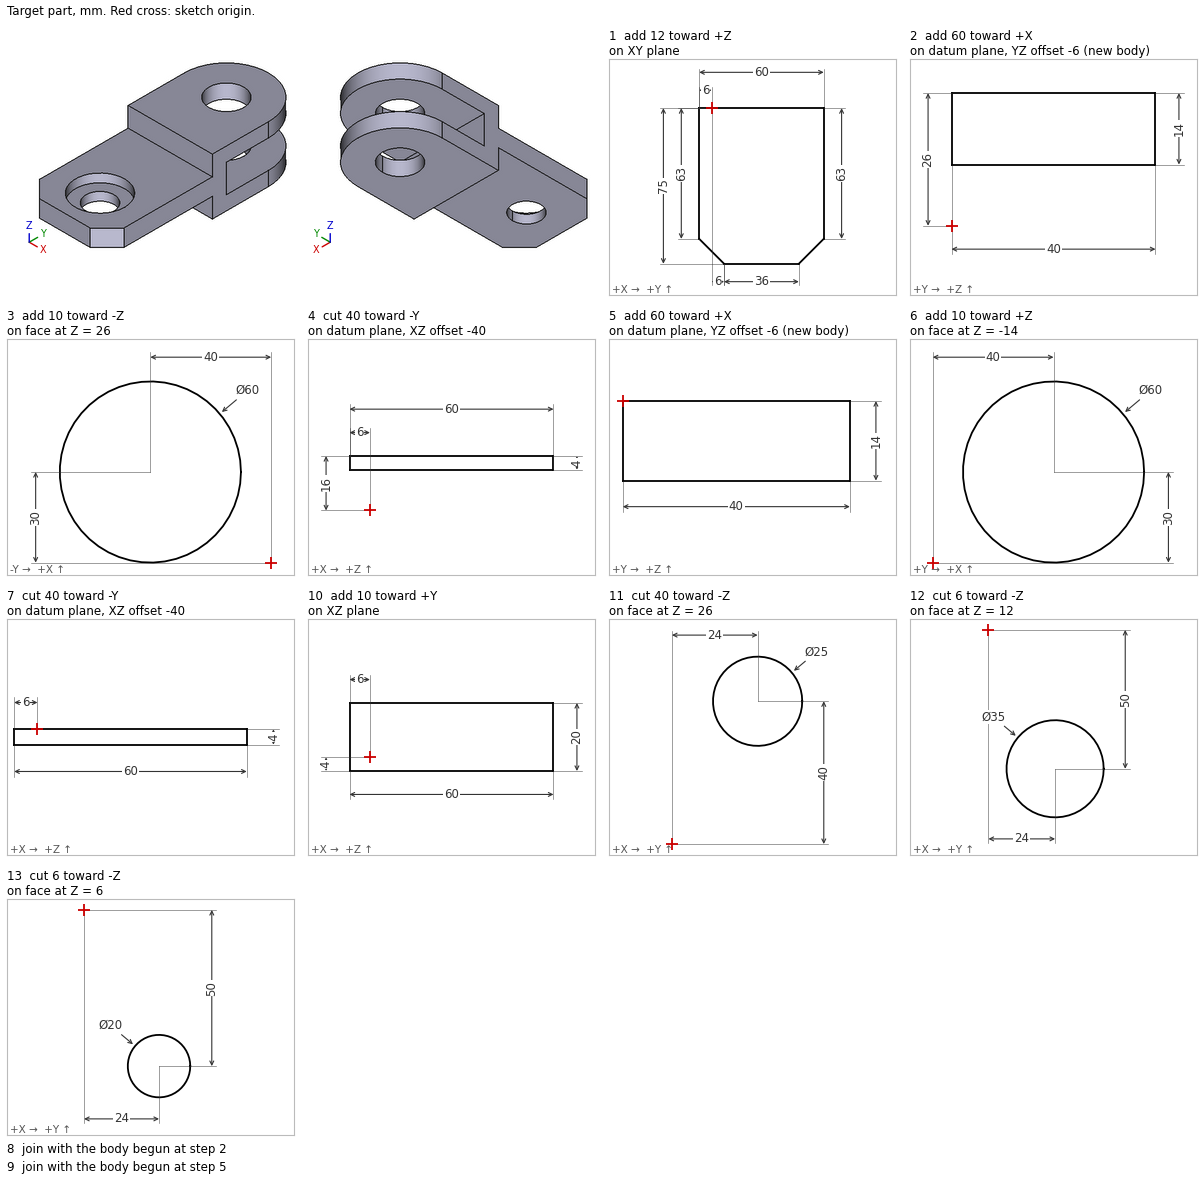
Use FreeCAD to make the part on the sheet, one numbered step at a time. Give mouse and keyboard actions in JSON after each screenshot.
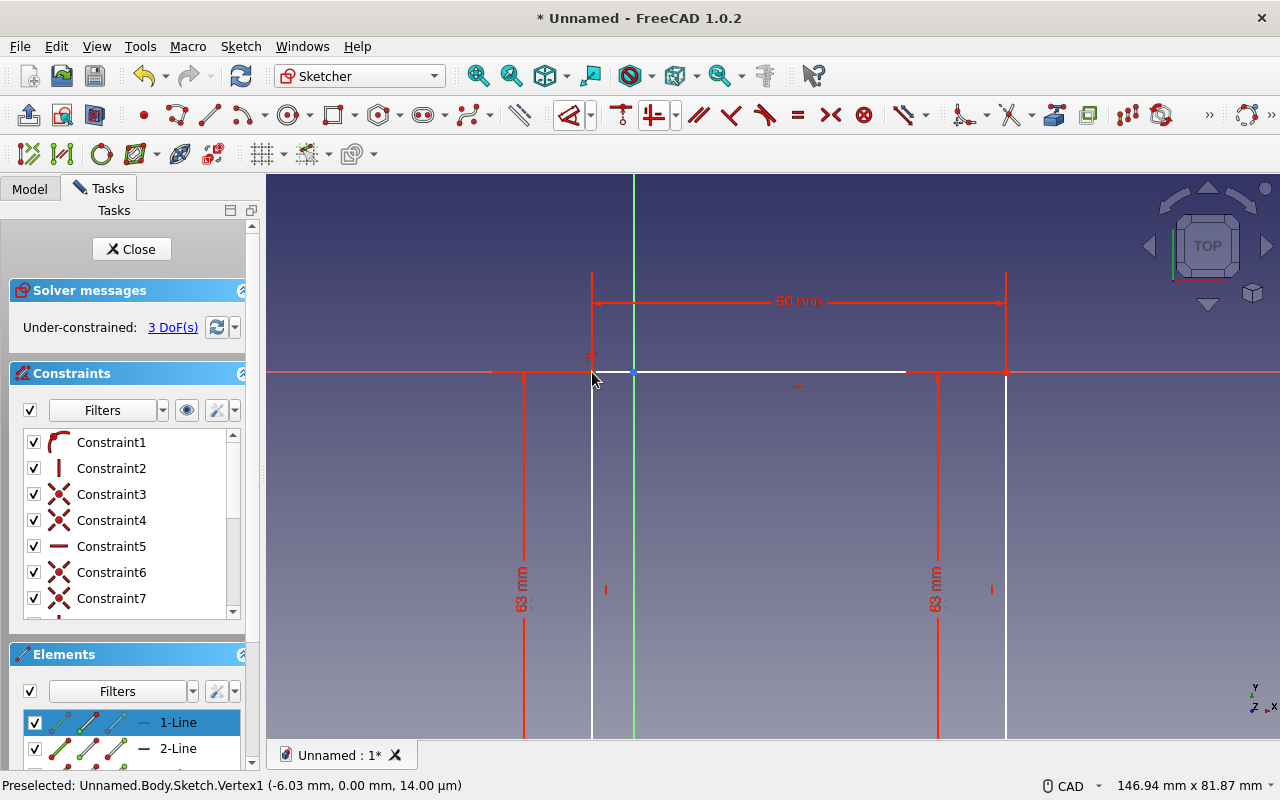
{"action": "left_click", "coordinate": [590, 116]}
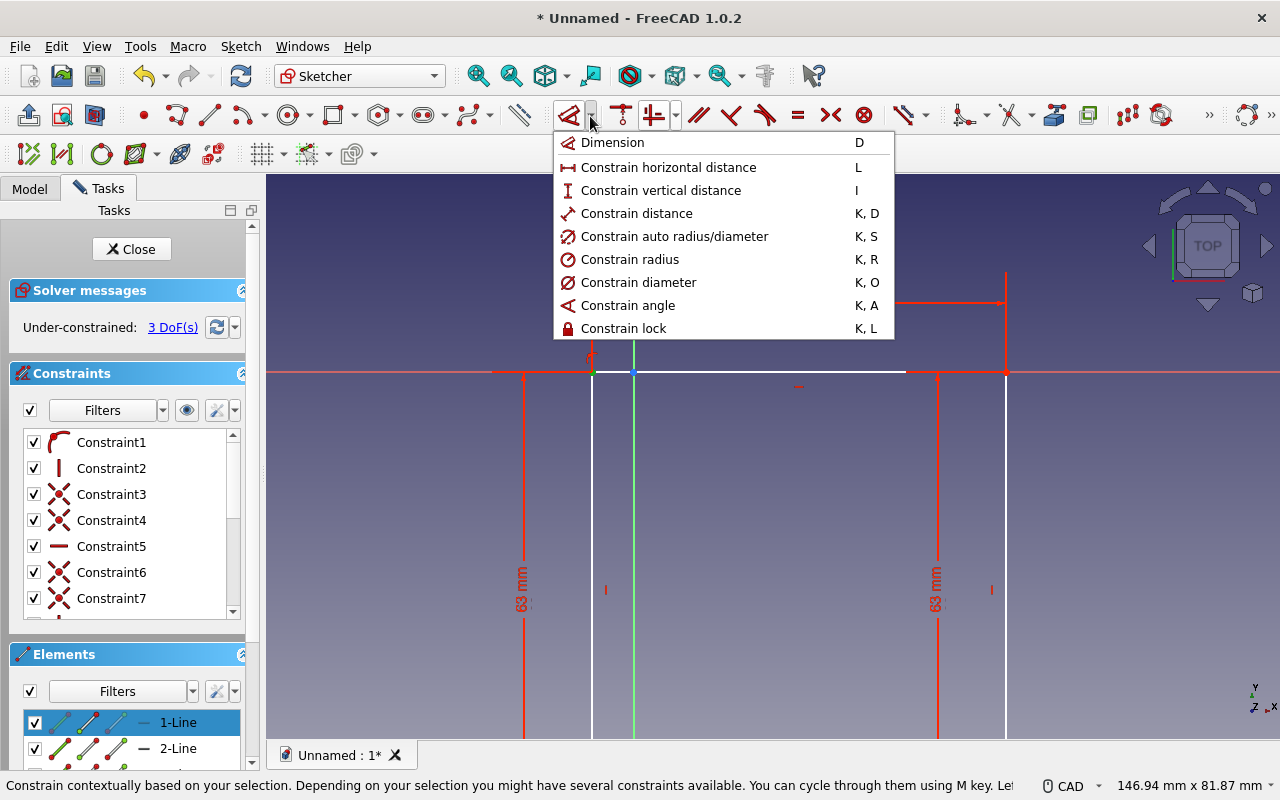
{"action": "left_click", "coordinate": [724, 168]}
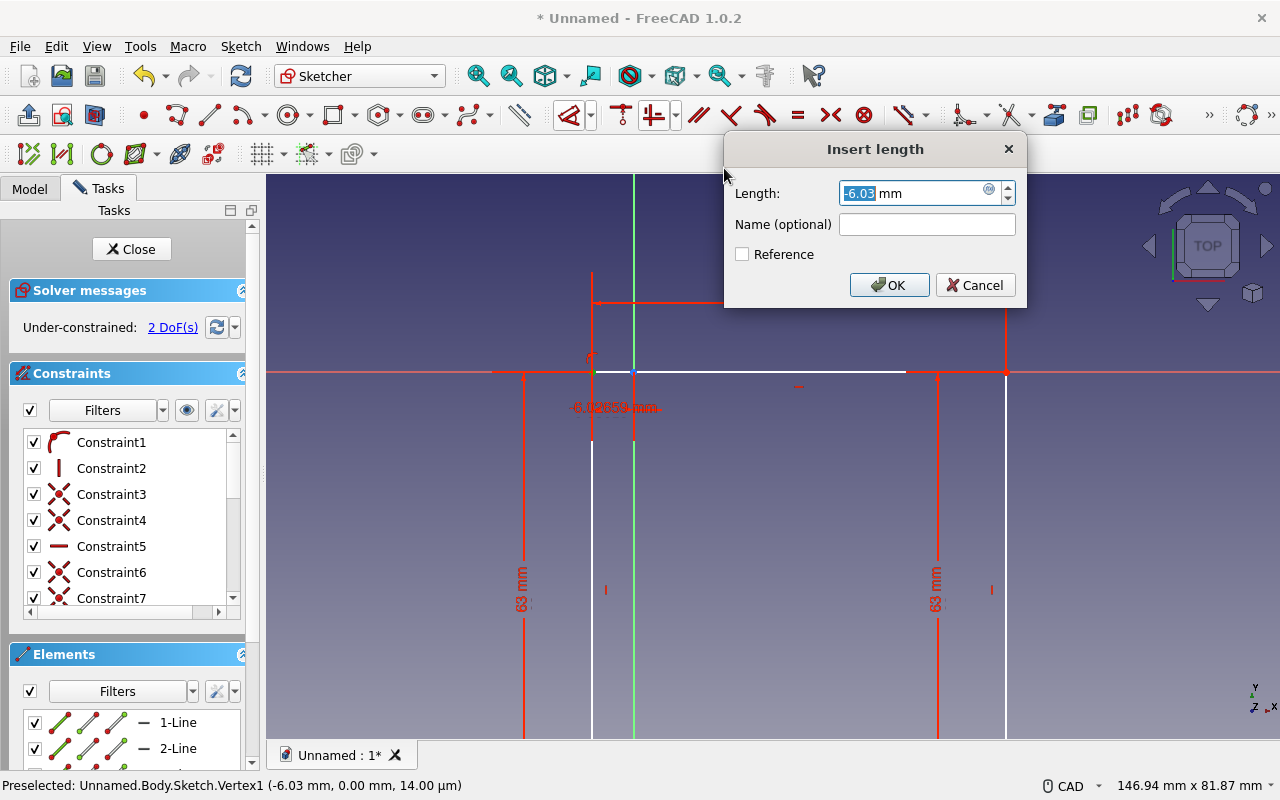
{"action": "type", "text": "-6"}
{"action": "key", "text": "Return"}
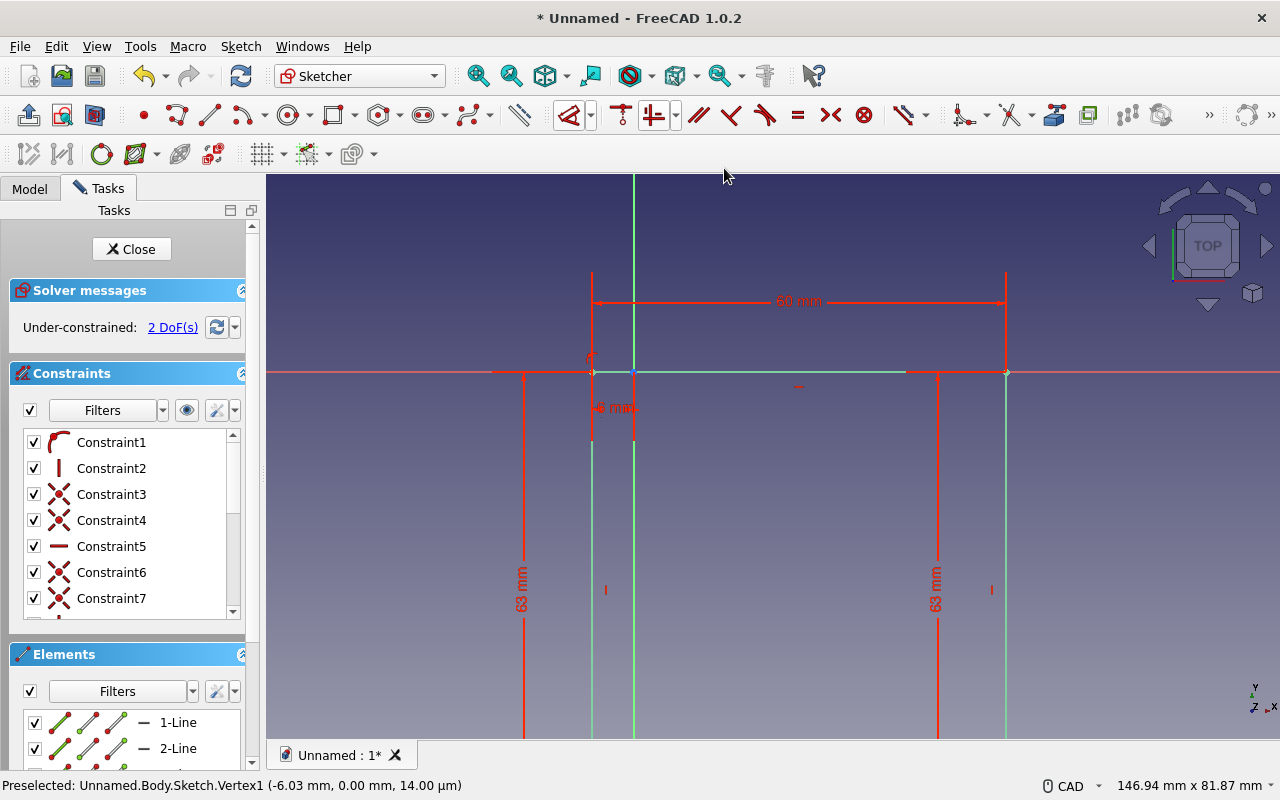
{"action": "scroll", "coordinate": [511, 202], "scroll_direction": "down", "scroll_amount": 2}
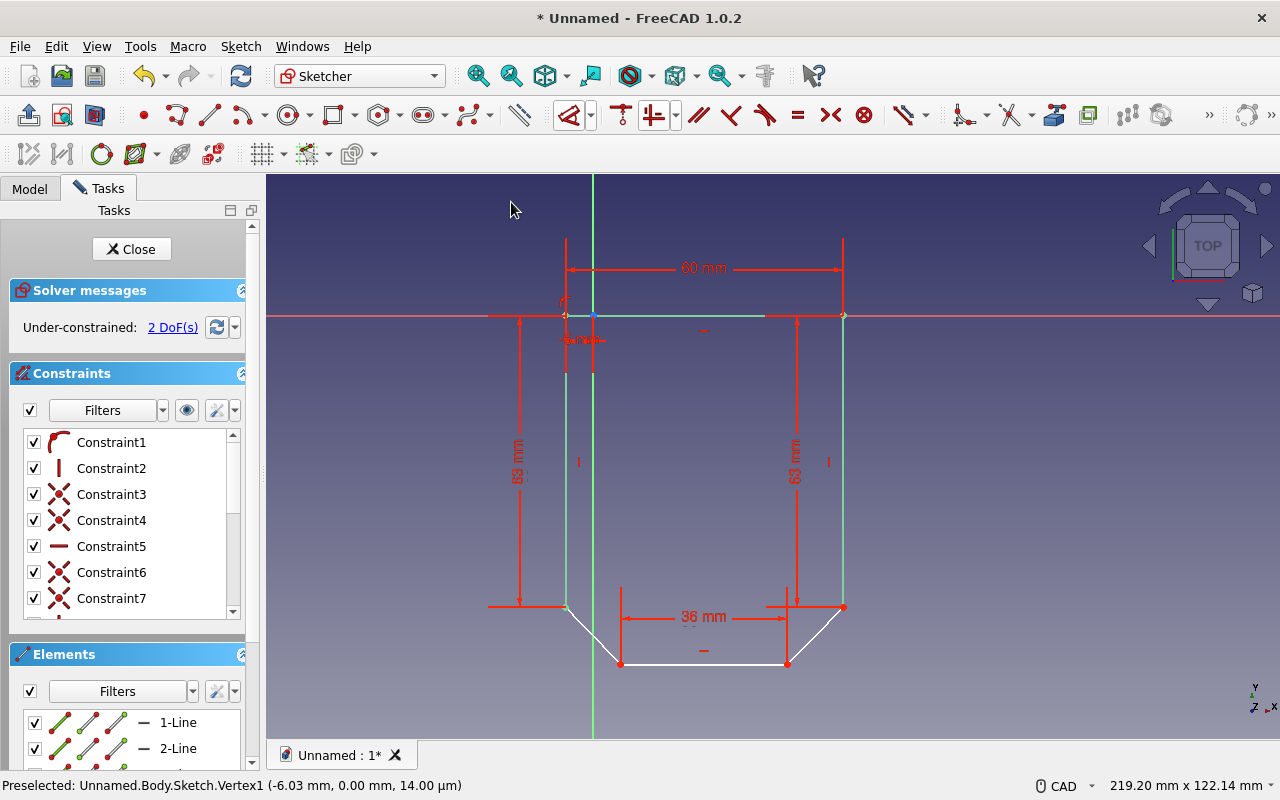
{"action": "scroll", "coordinate": [621, 665], "scroll_direction": "up", "scroll_amount": 2}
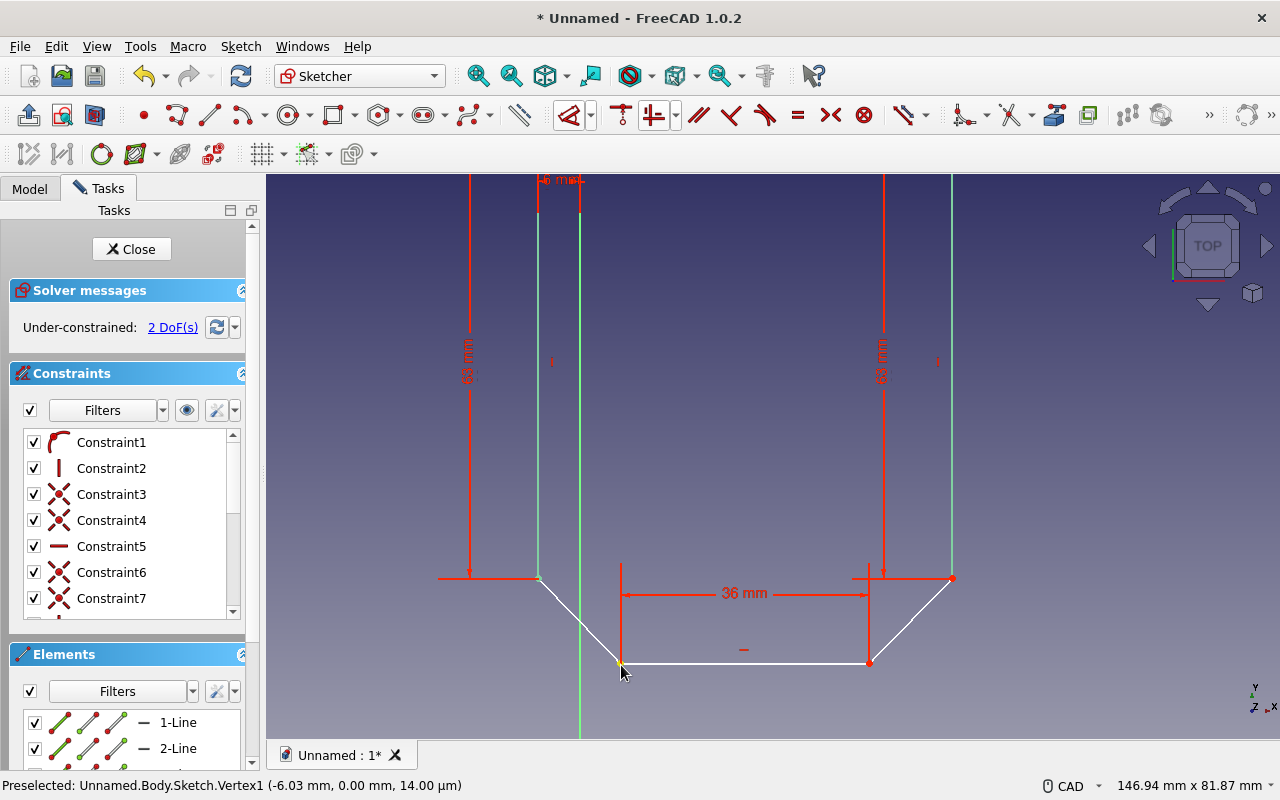
{"action": "left_click", "coordinate": [621, 664]}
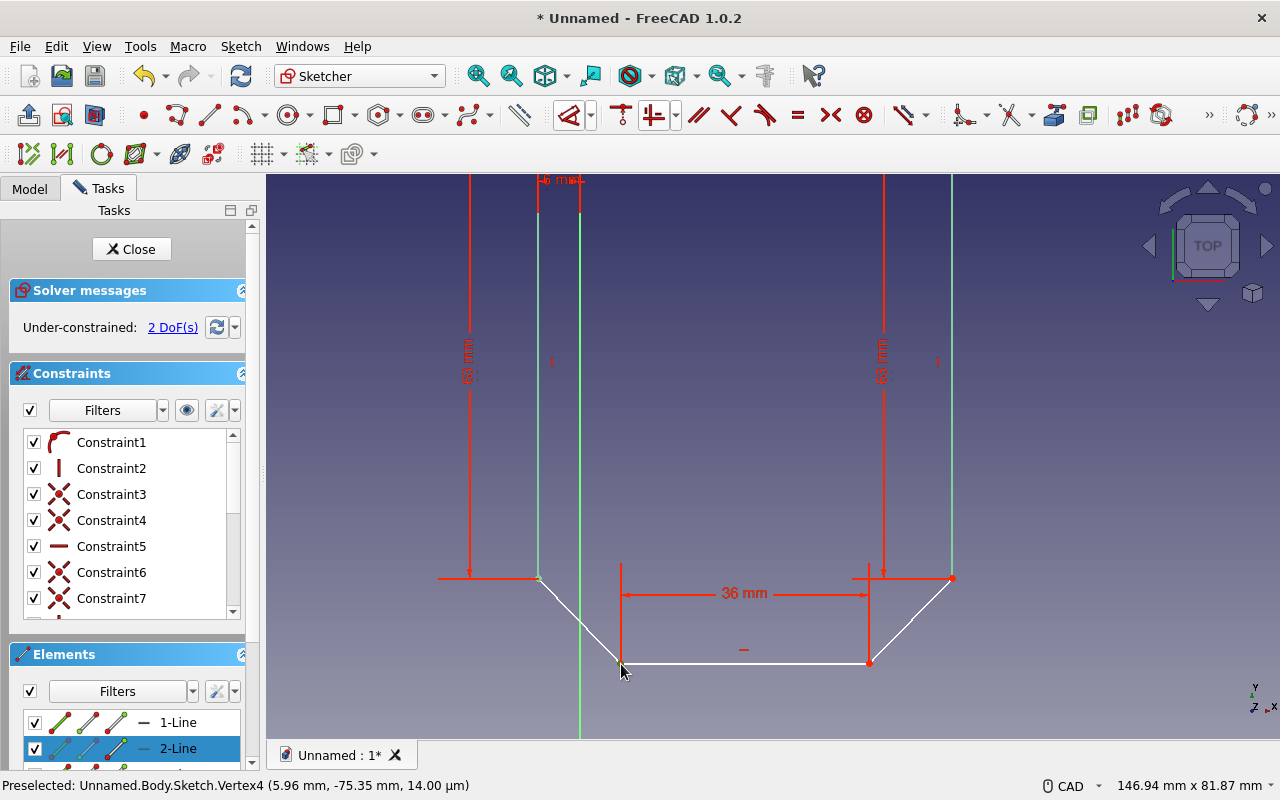
{"action": "key", "text": "l"}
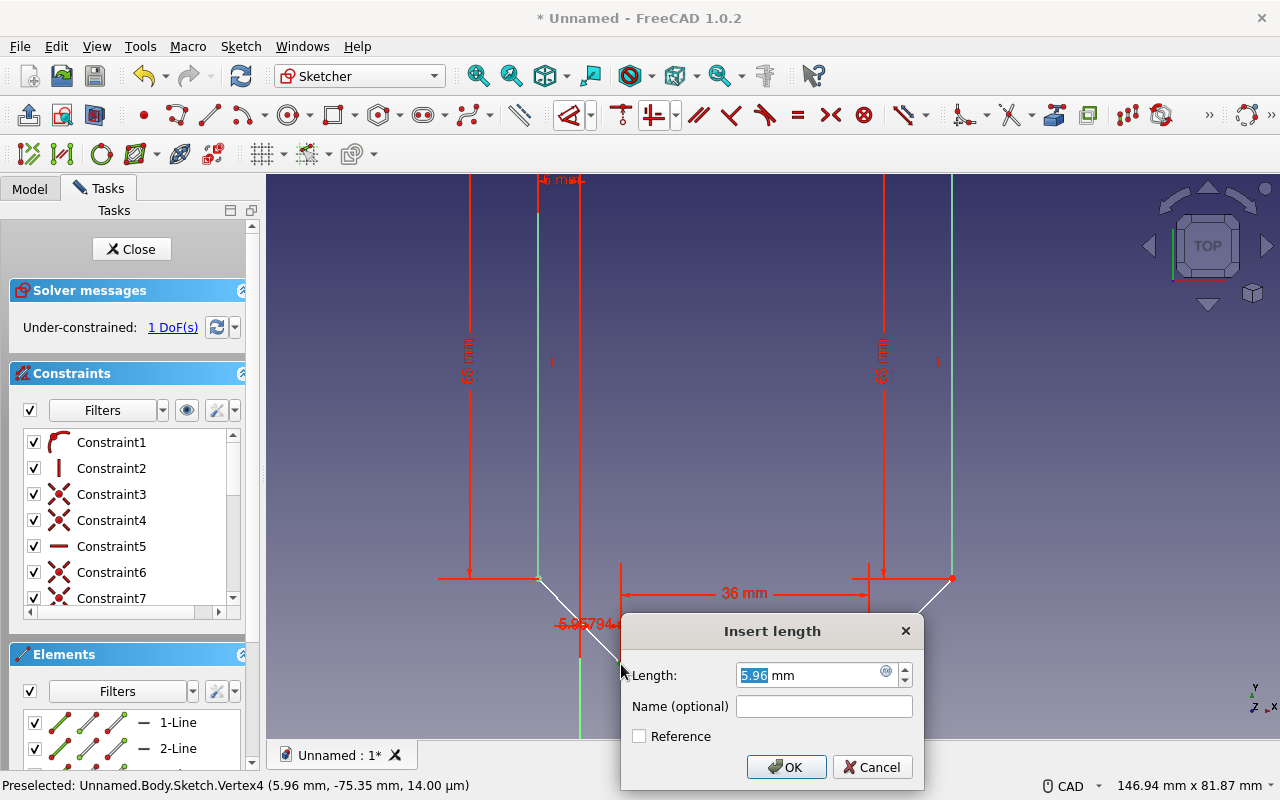
{"action": "type", "text": "6"}
{"action": "key", "text": "Return"}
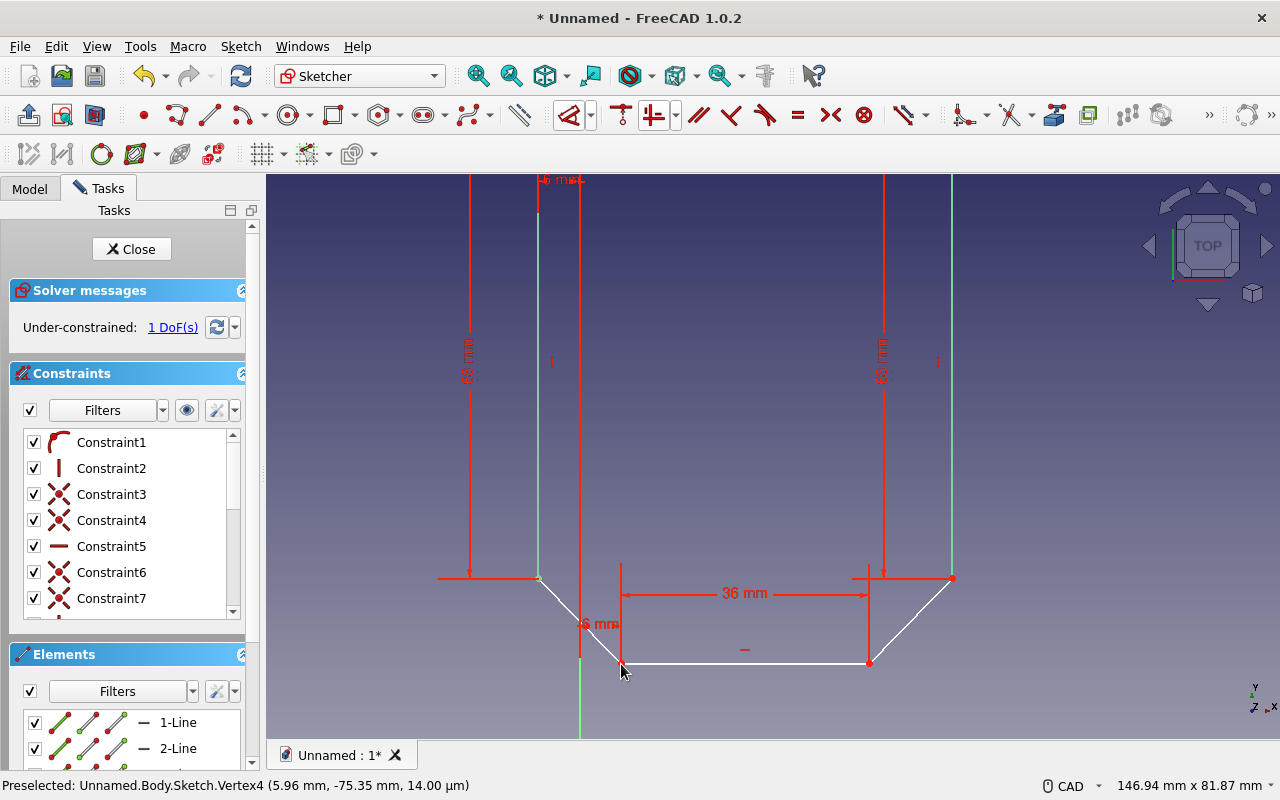
{"action": "left_click", "coordinate": [621, 664]}